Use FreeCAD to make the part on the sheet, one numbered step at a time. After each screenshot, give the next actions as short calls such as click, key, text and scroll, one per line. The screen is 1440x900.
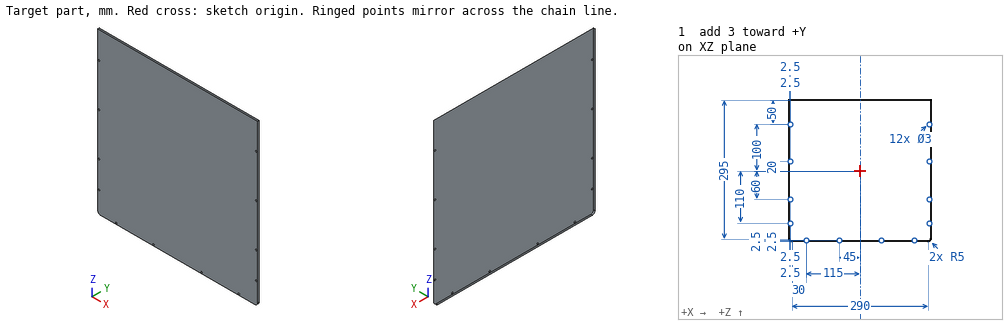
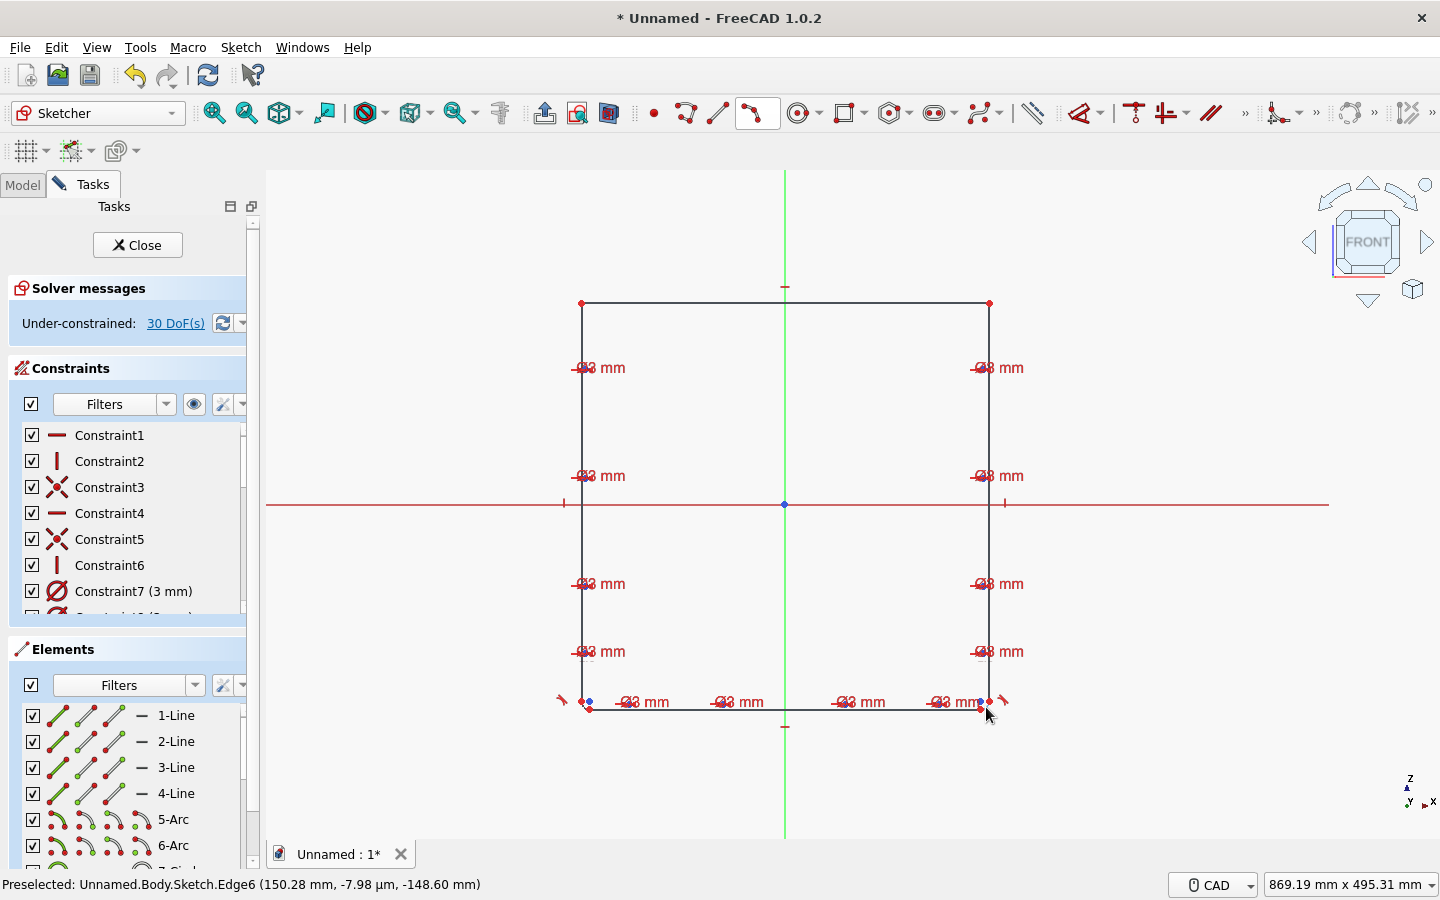
scroll(584, 707, up, 4)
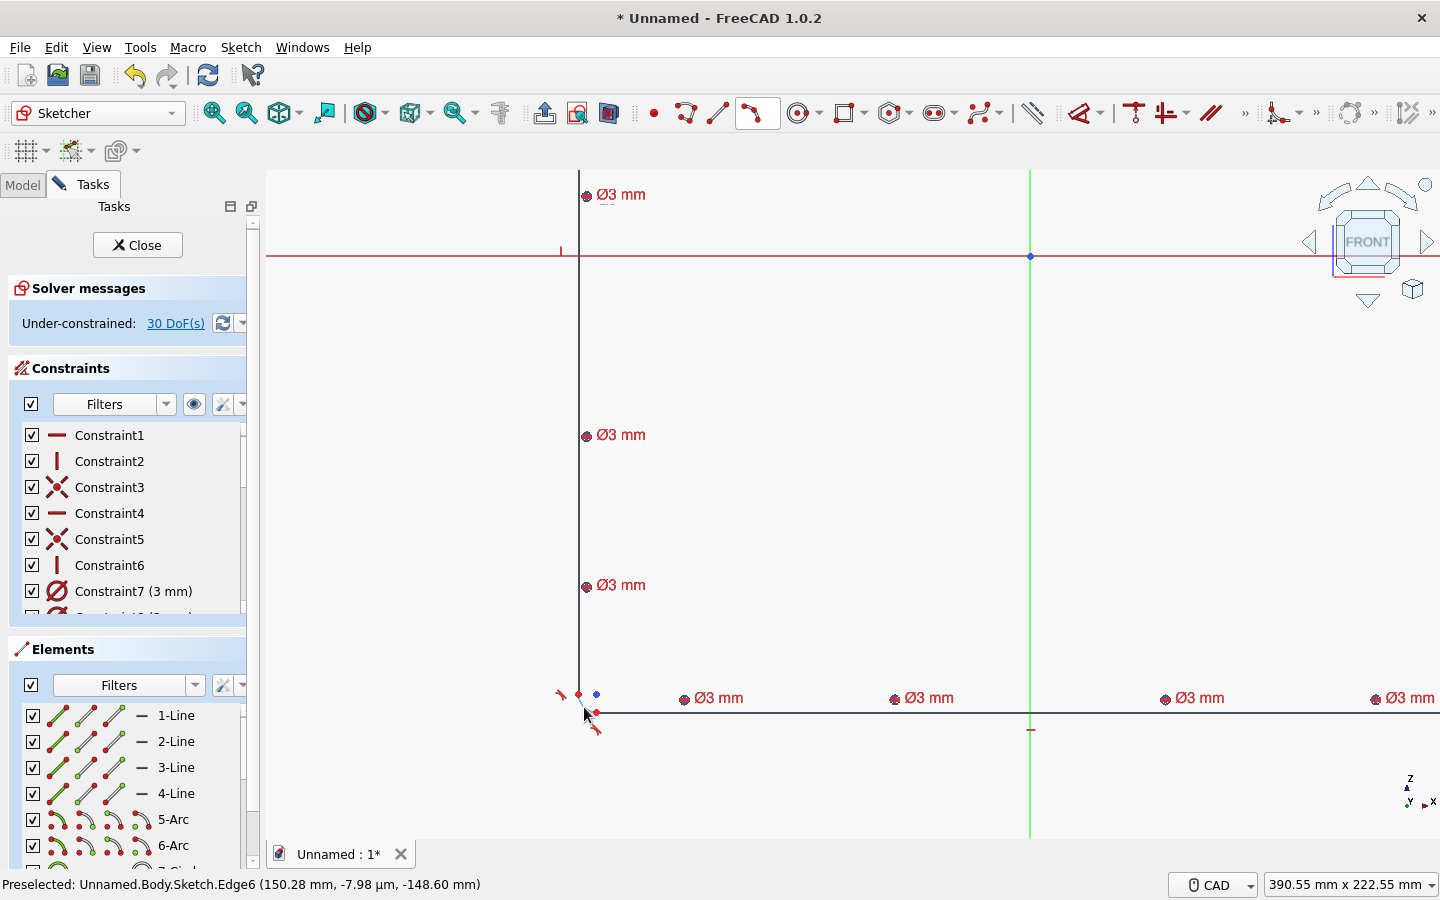
click(584, 707)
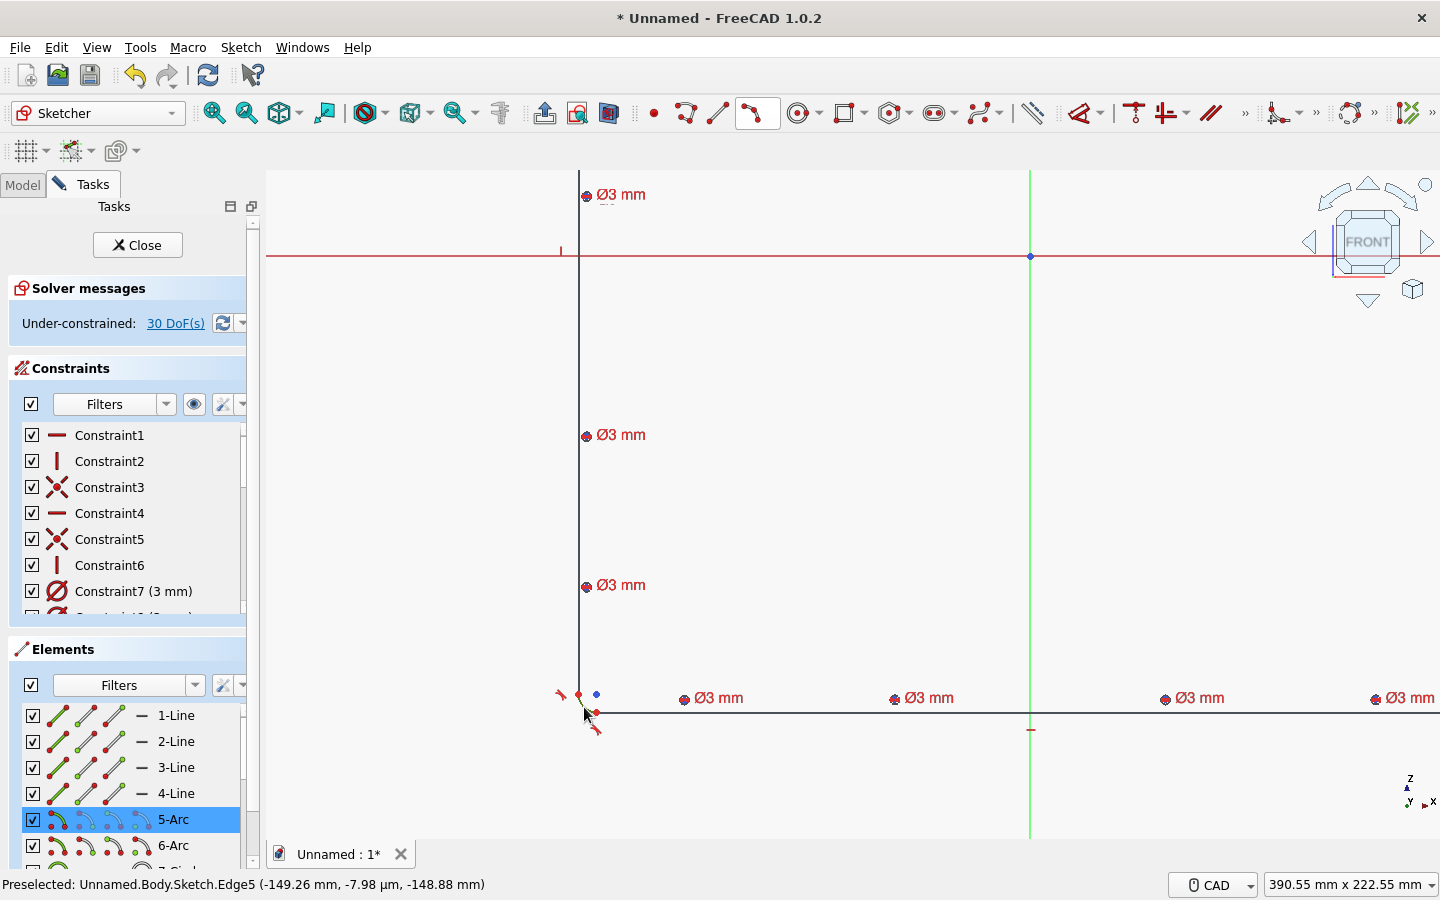
scroll(584, 707, down, 4)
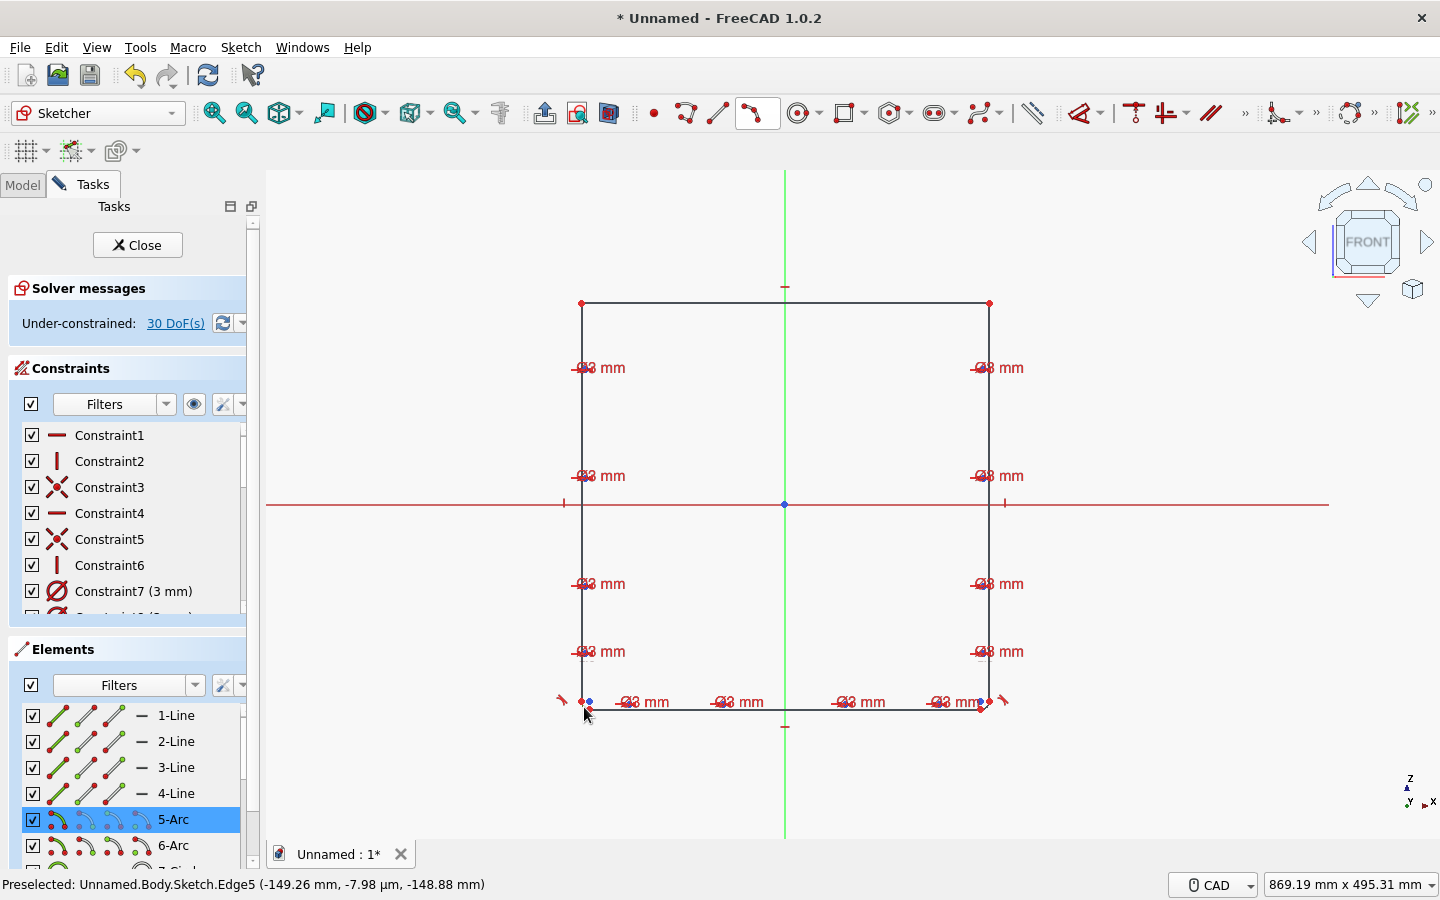
scroll(987, 707, up, 4)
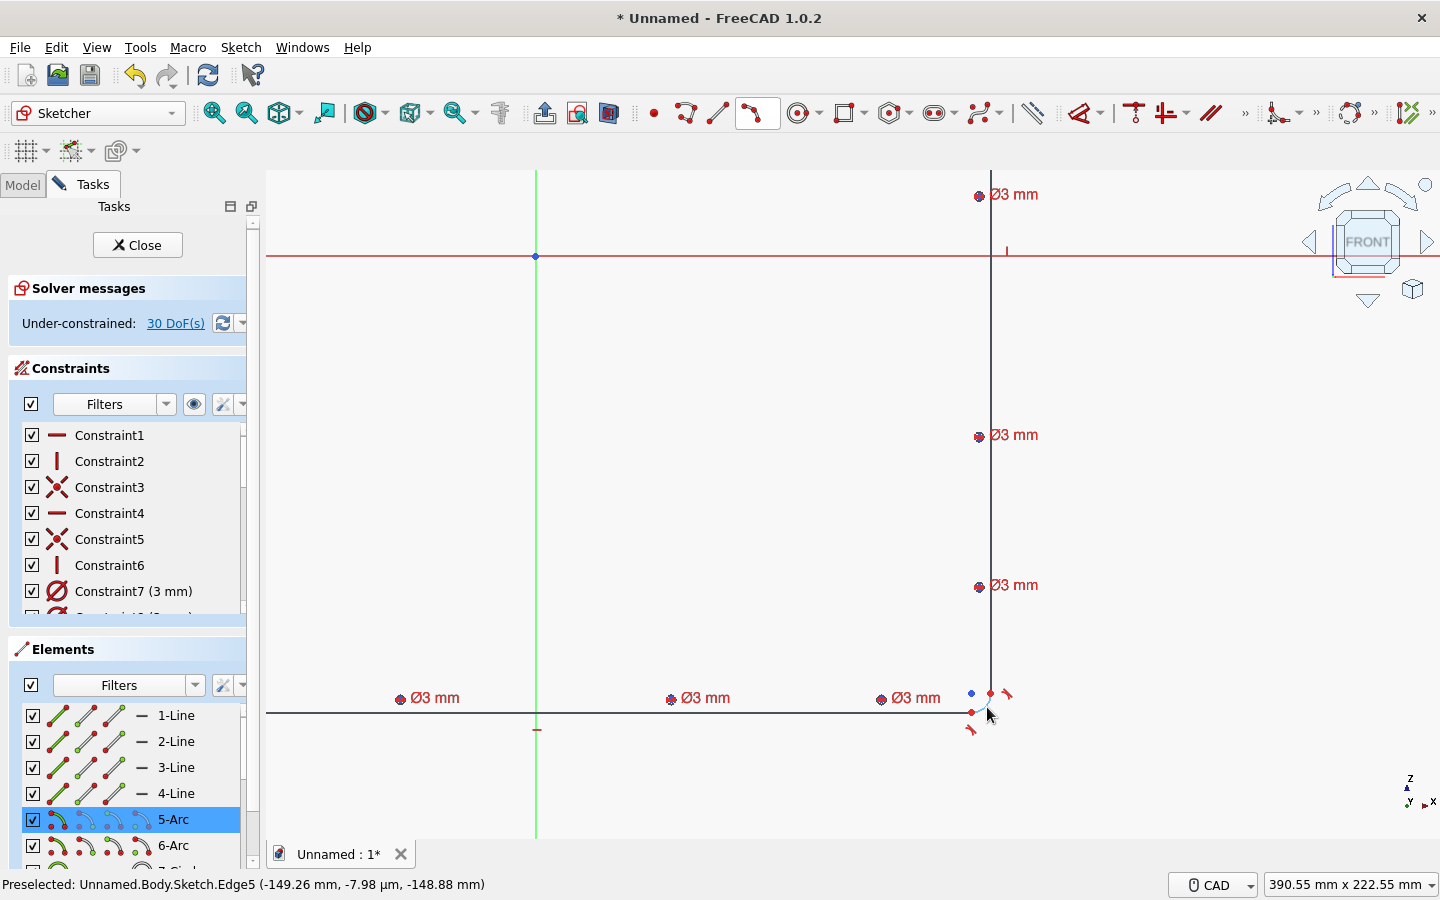
click(985, 707)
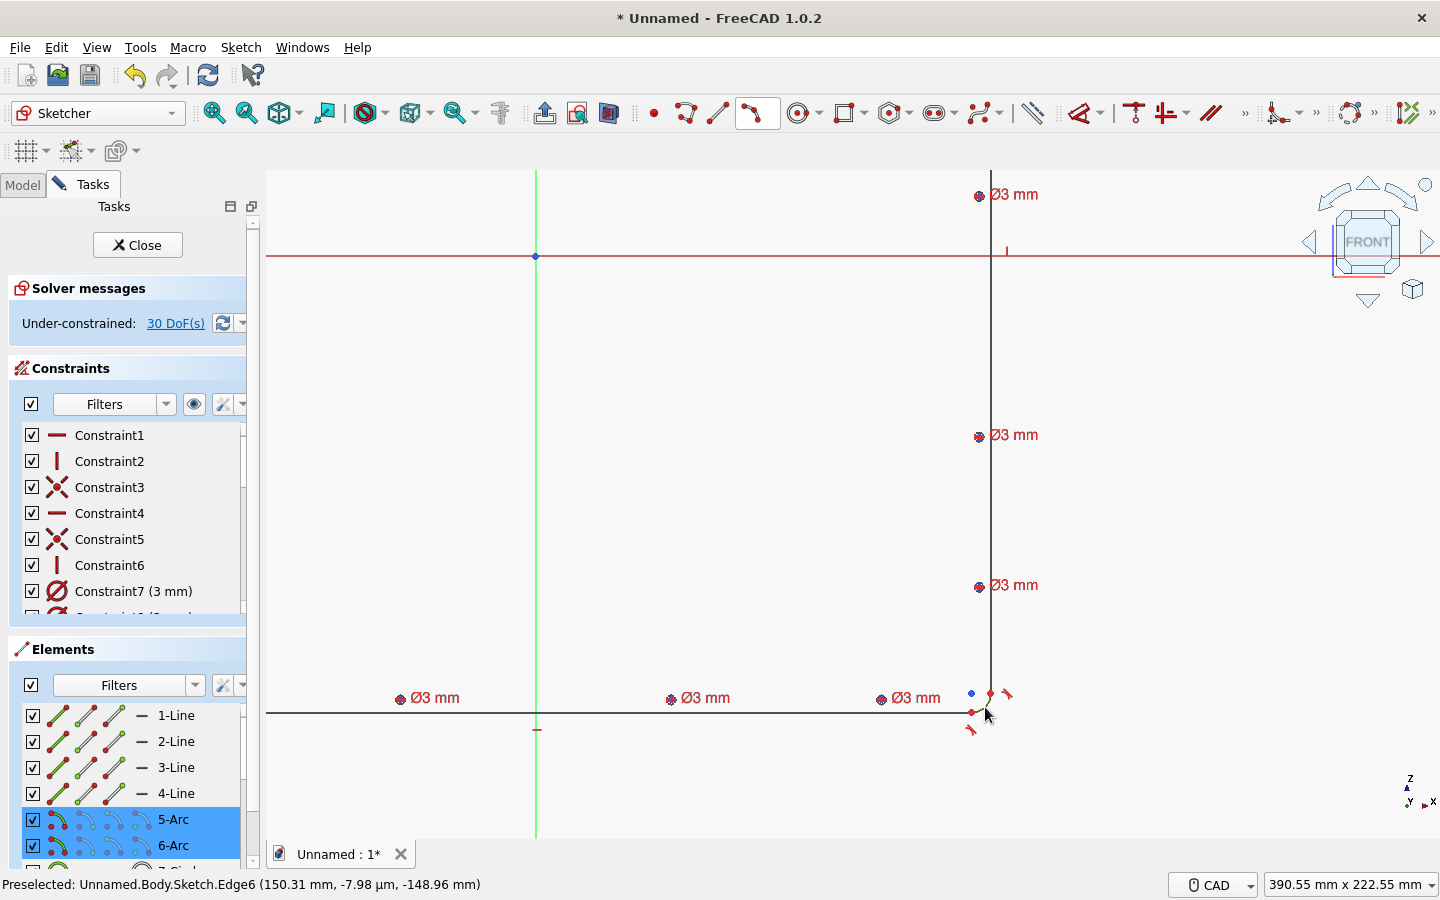
key(e)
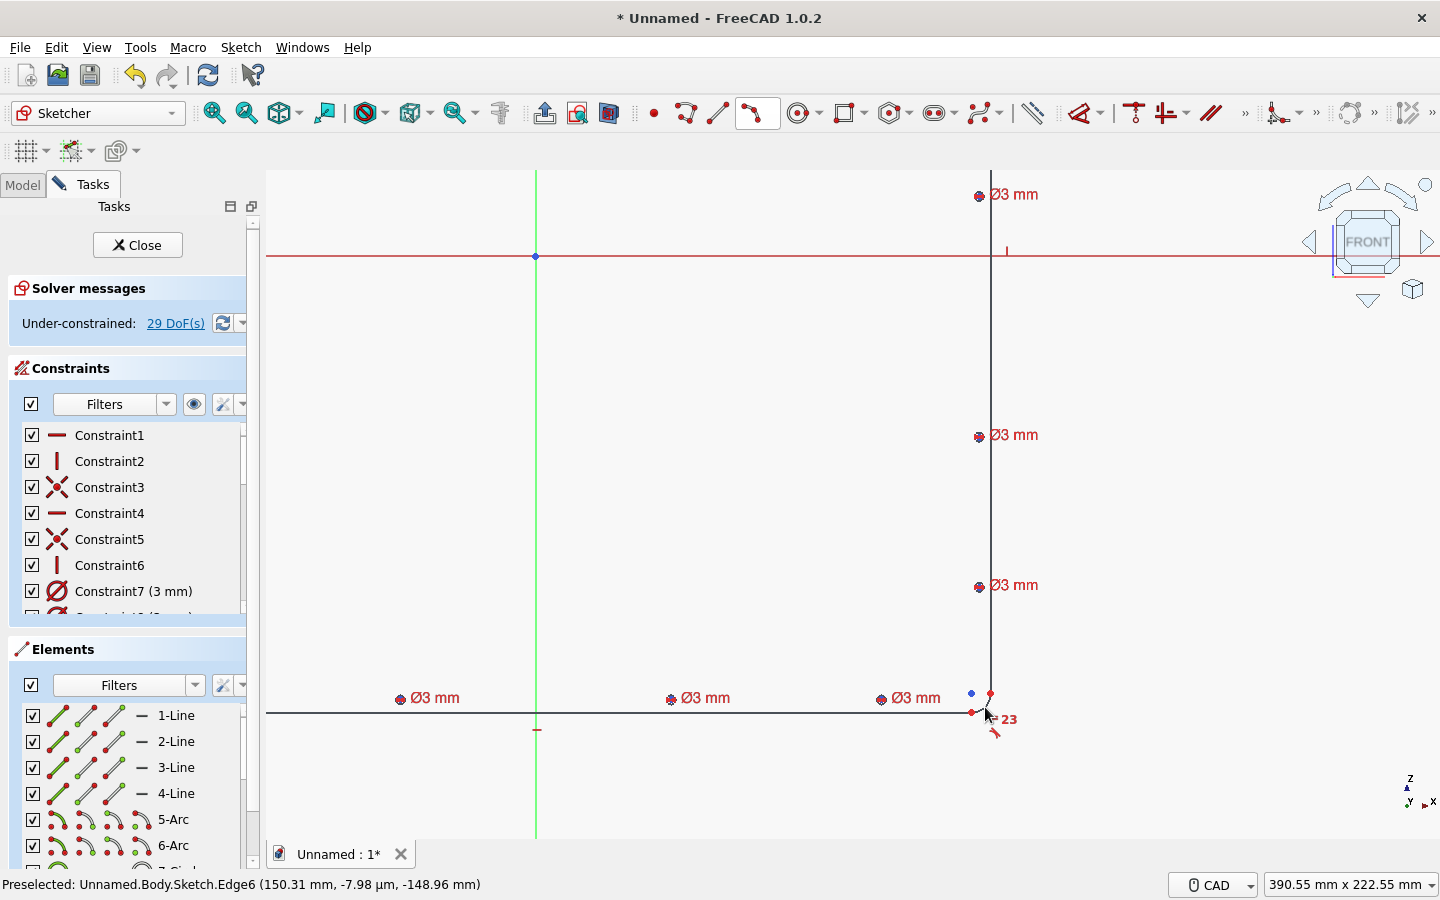
scroll(987, 707, down, 4)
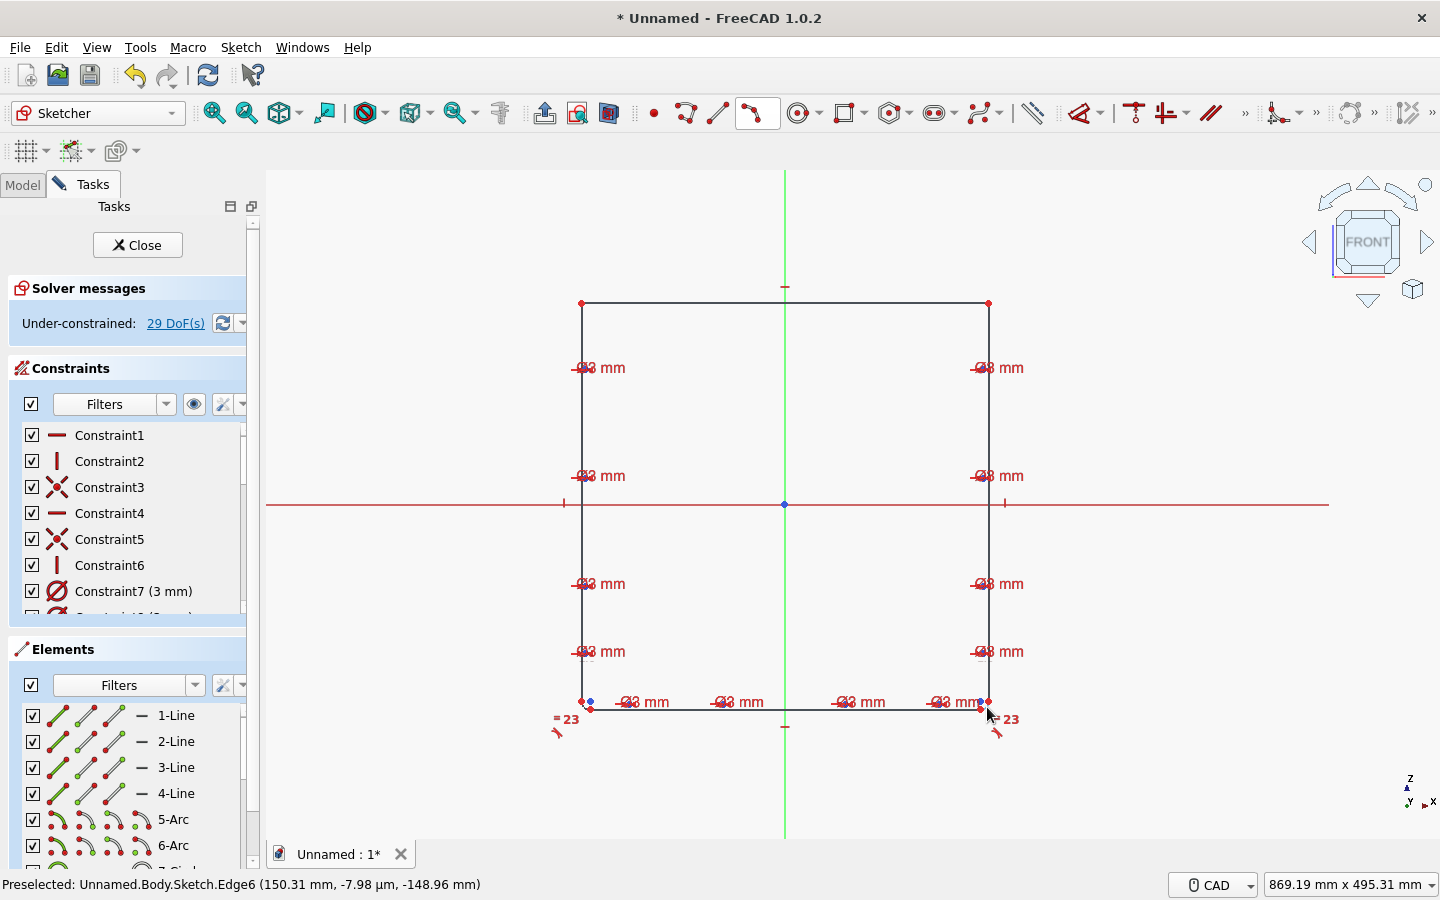
click(585, 370)